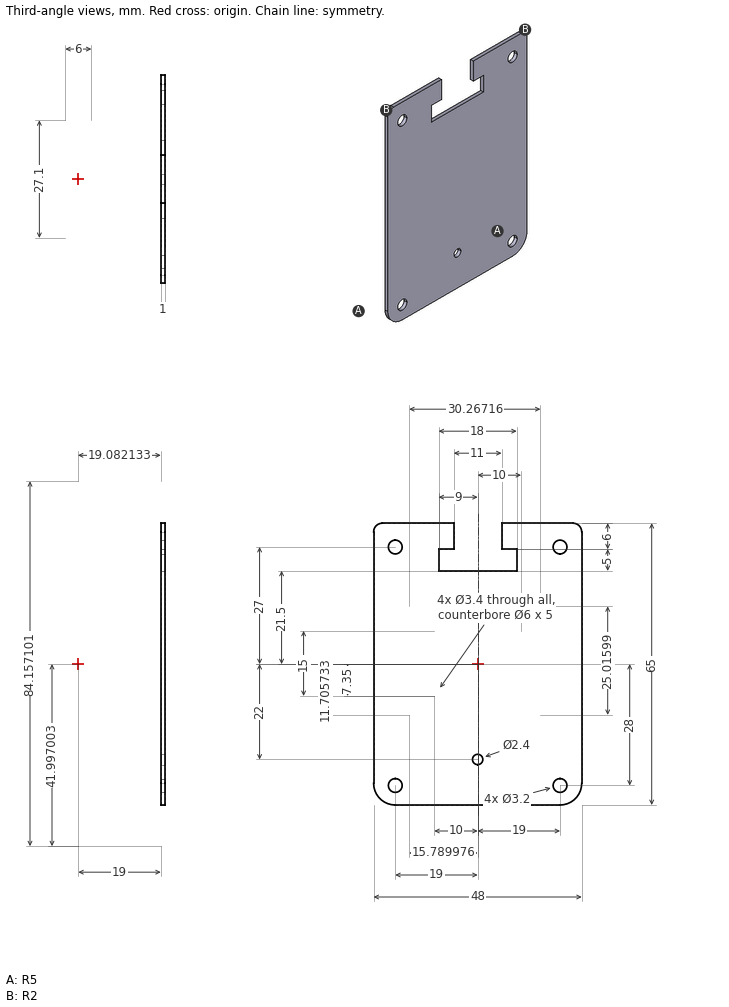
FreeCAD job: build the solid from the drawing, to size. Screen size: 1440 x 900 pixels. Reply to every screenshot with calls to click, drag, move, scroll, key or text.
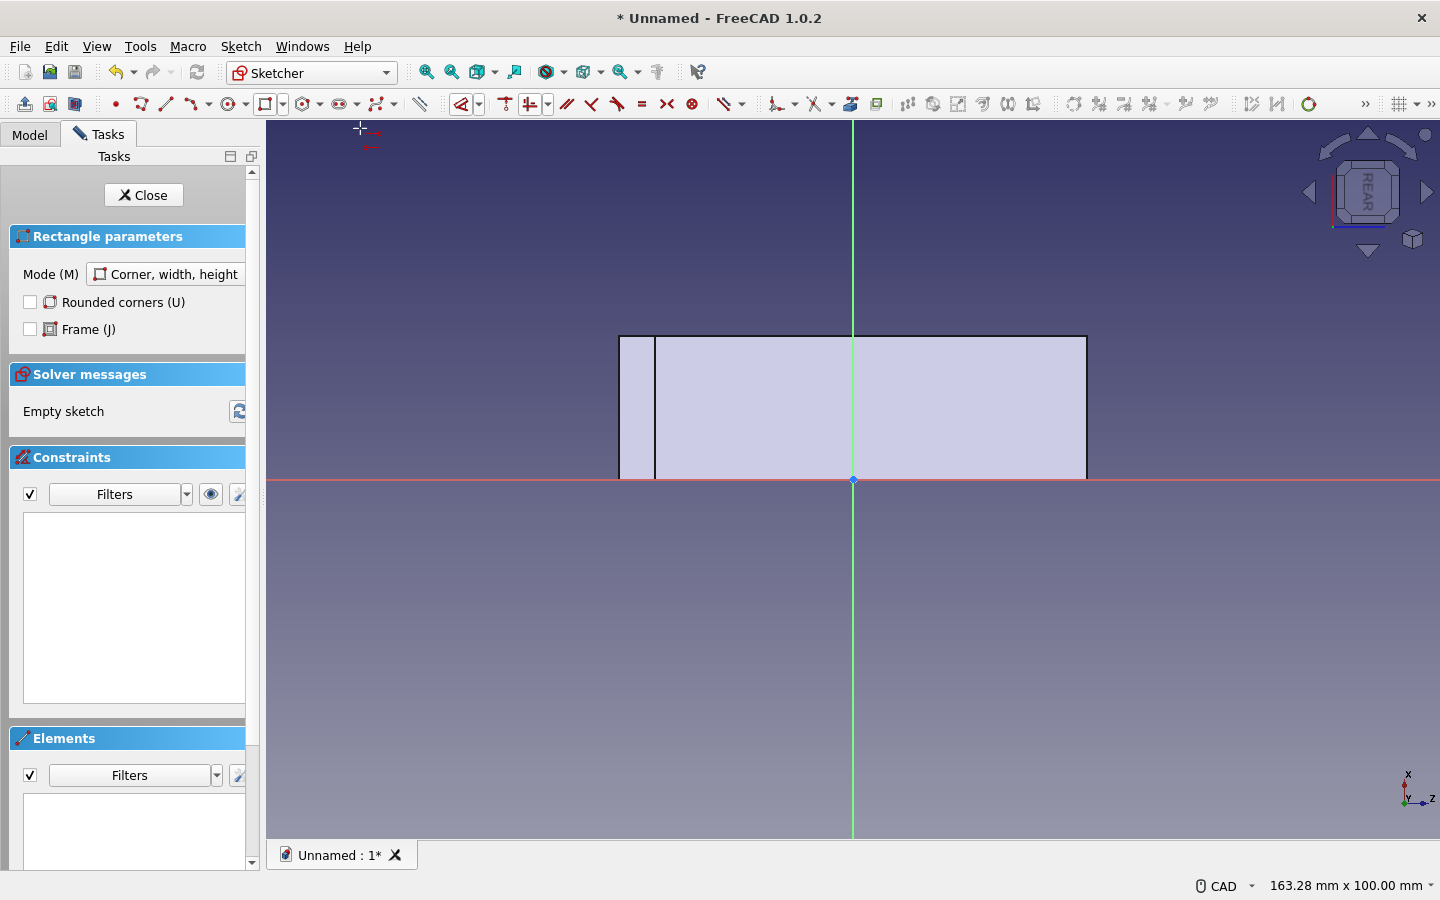
click(551, 343)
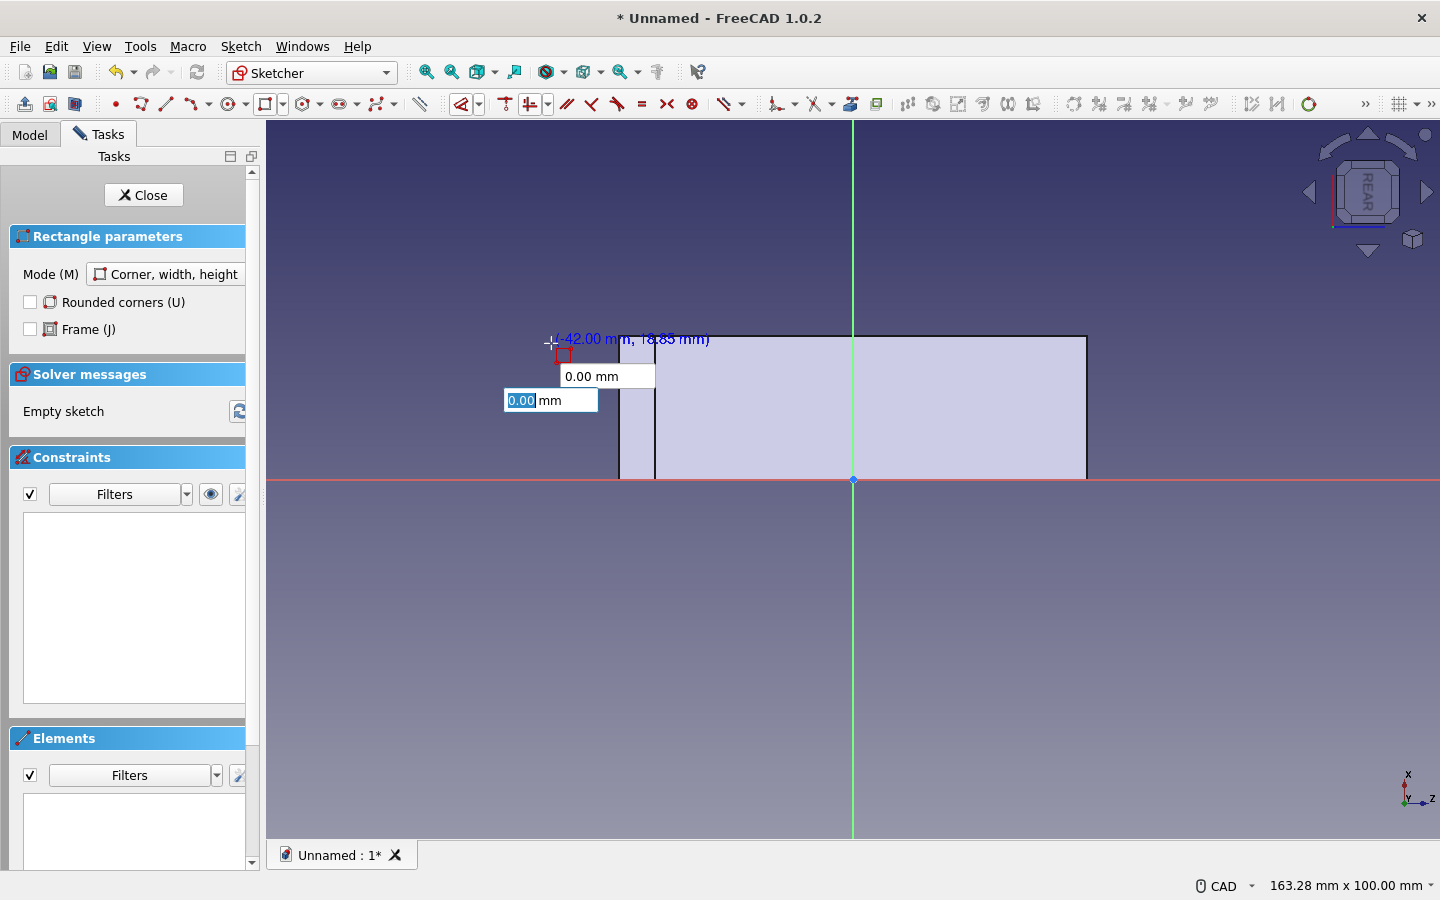
scroll(1156, 480, up, 17)
move(1138, 468)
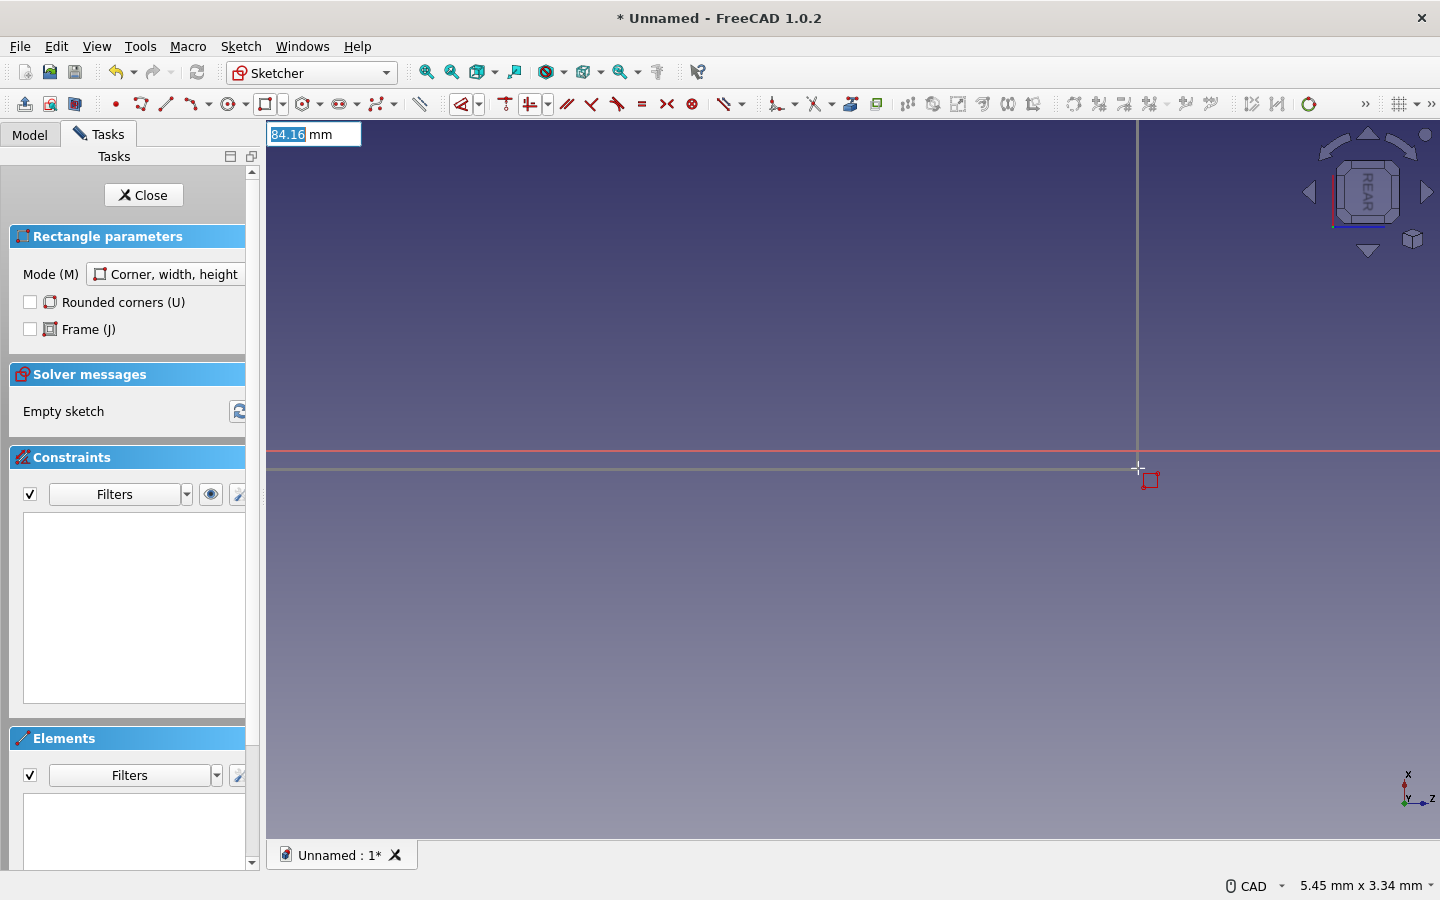
text(84.157101)
key(Tab)
text(19.082133)
key(Return)
key(Escape)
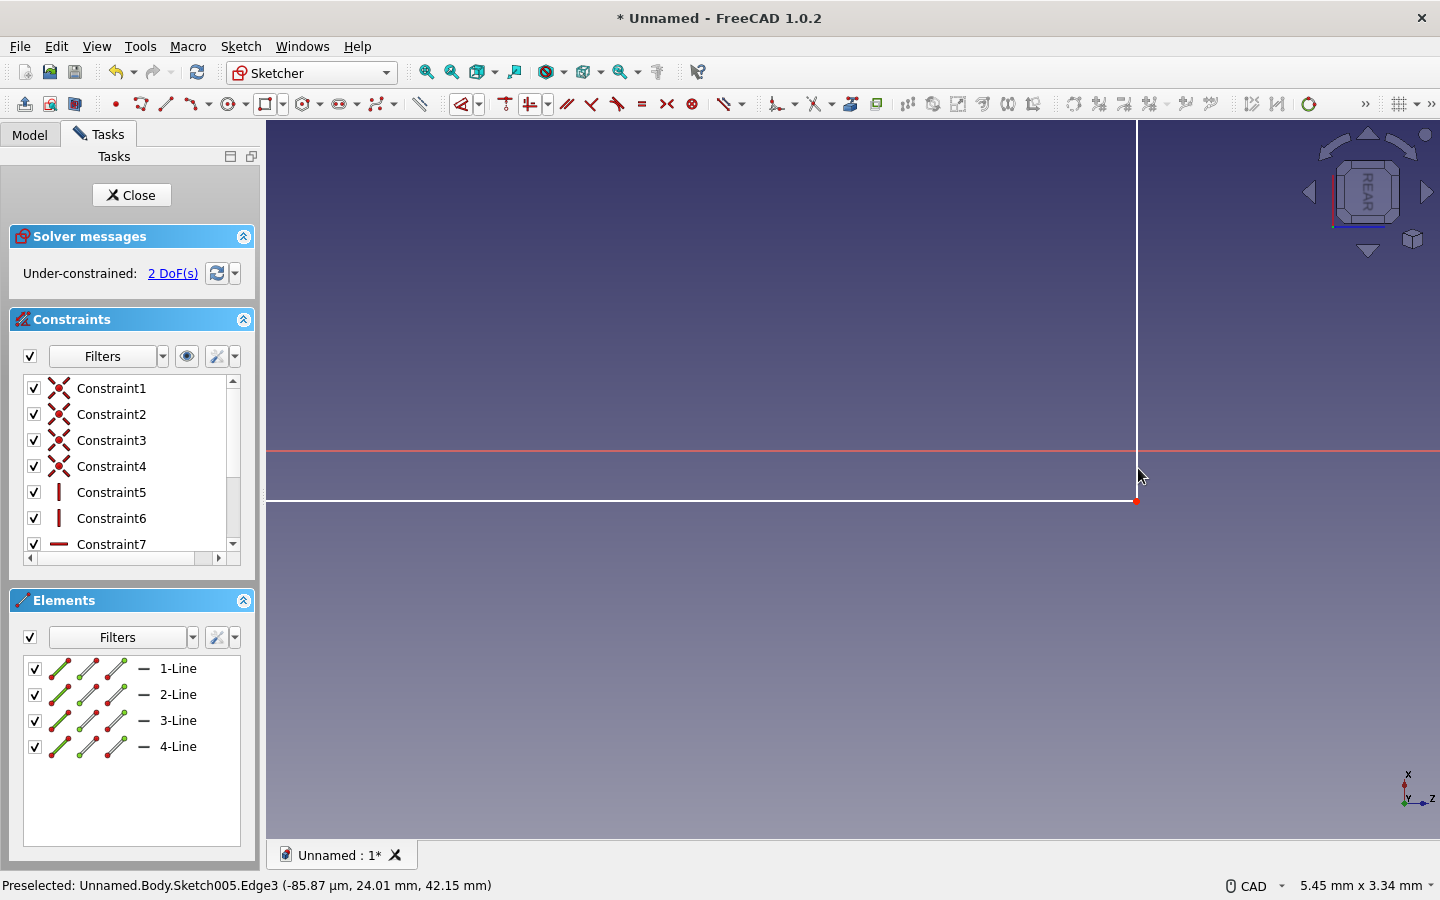
scroll(1241, 588, down, 15)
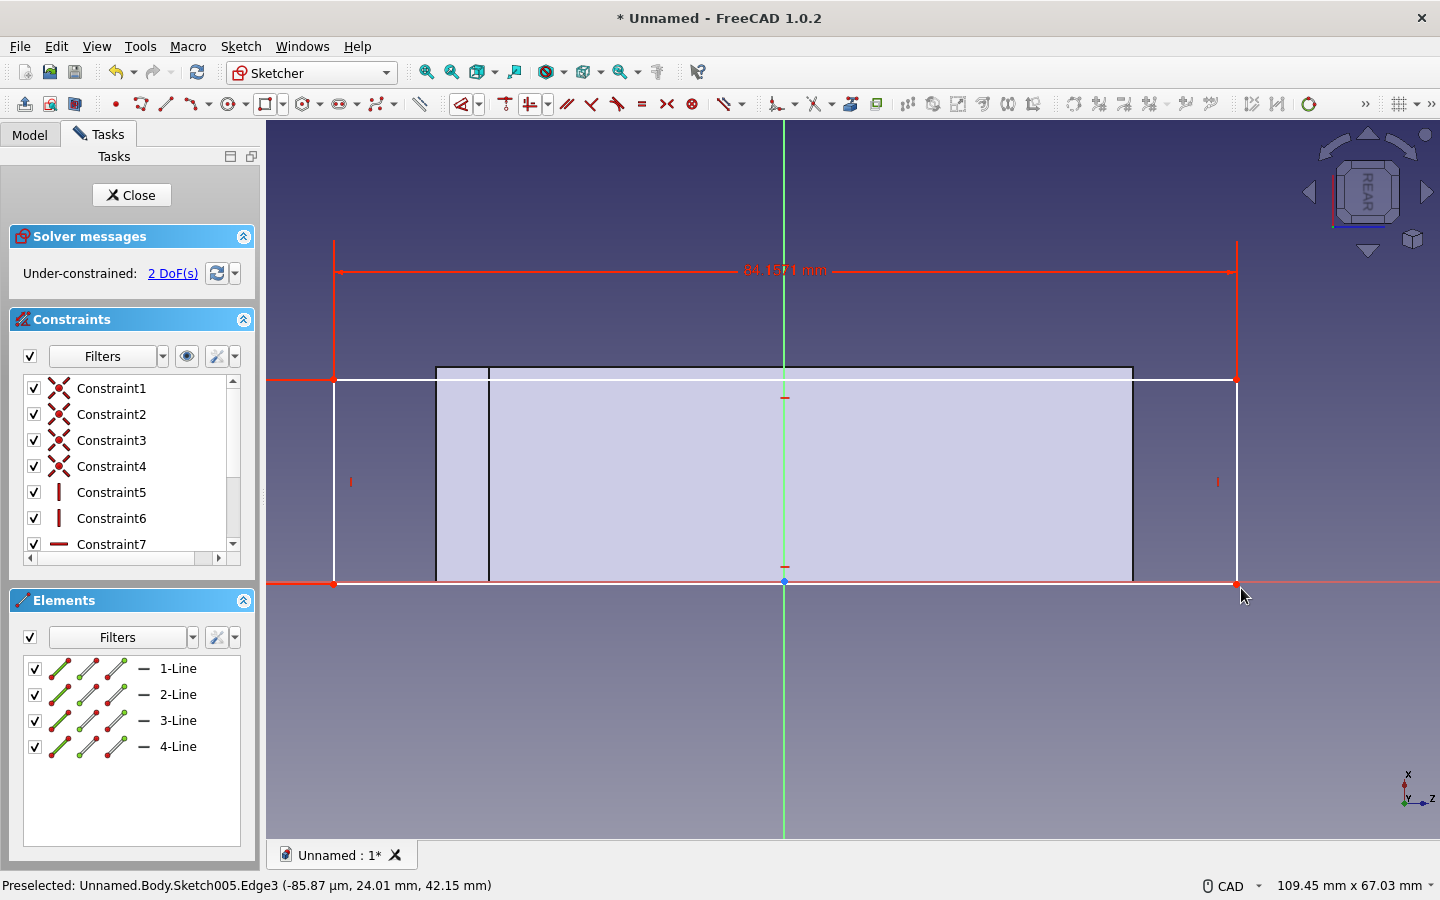
click(334, 380)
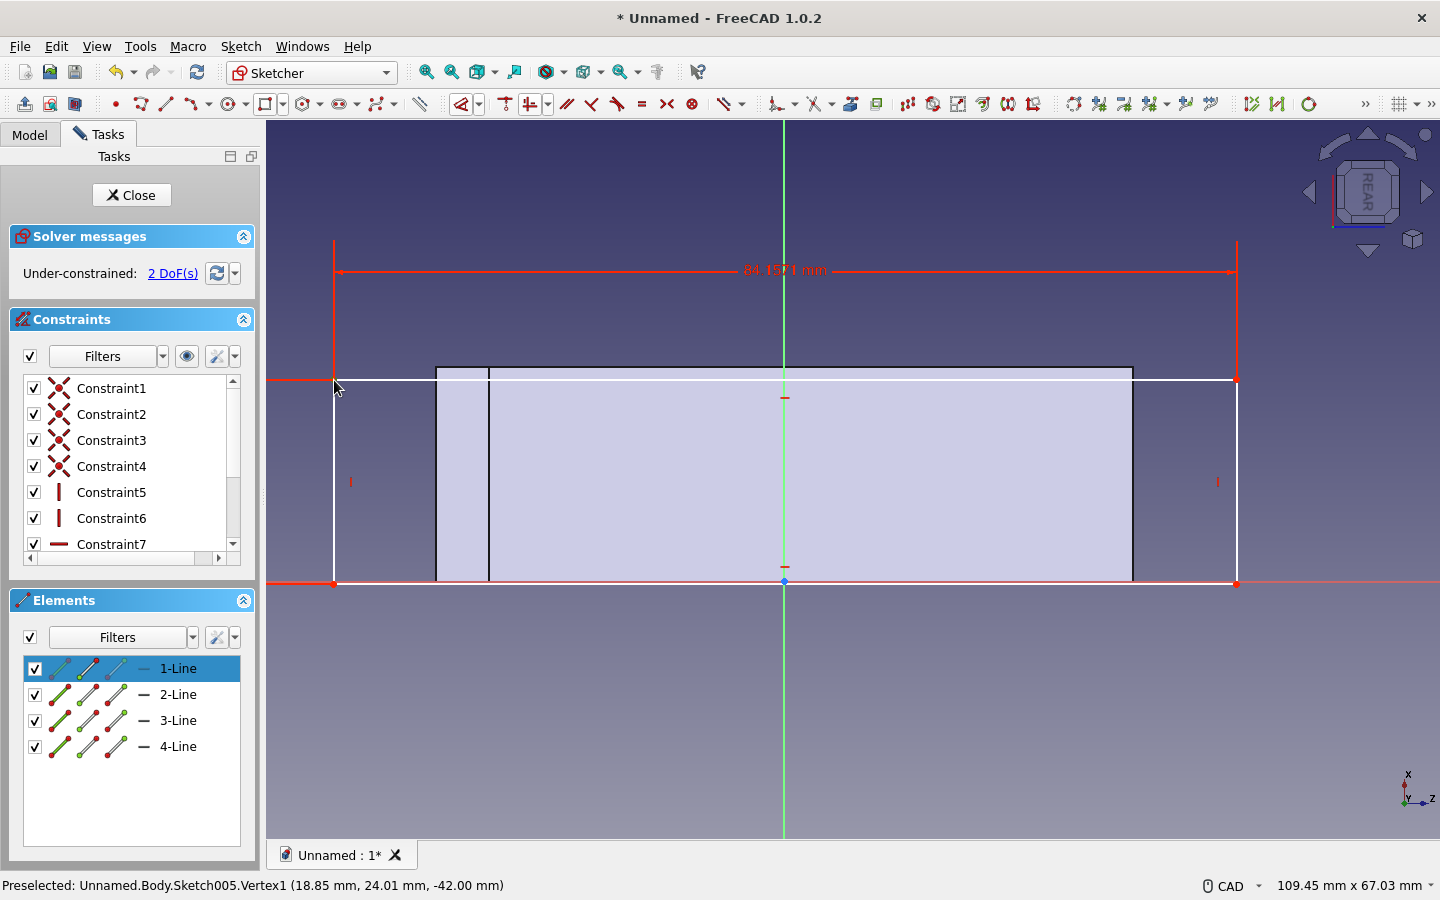
key(i)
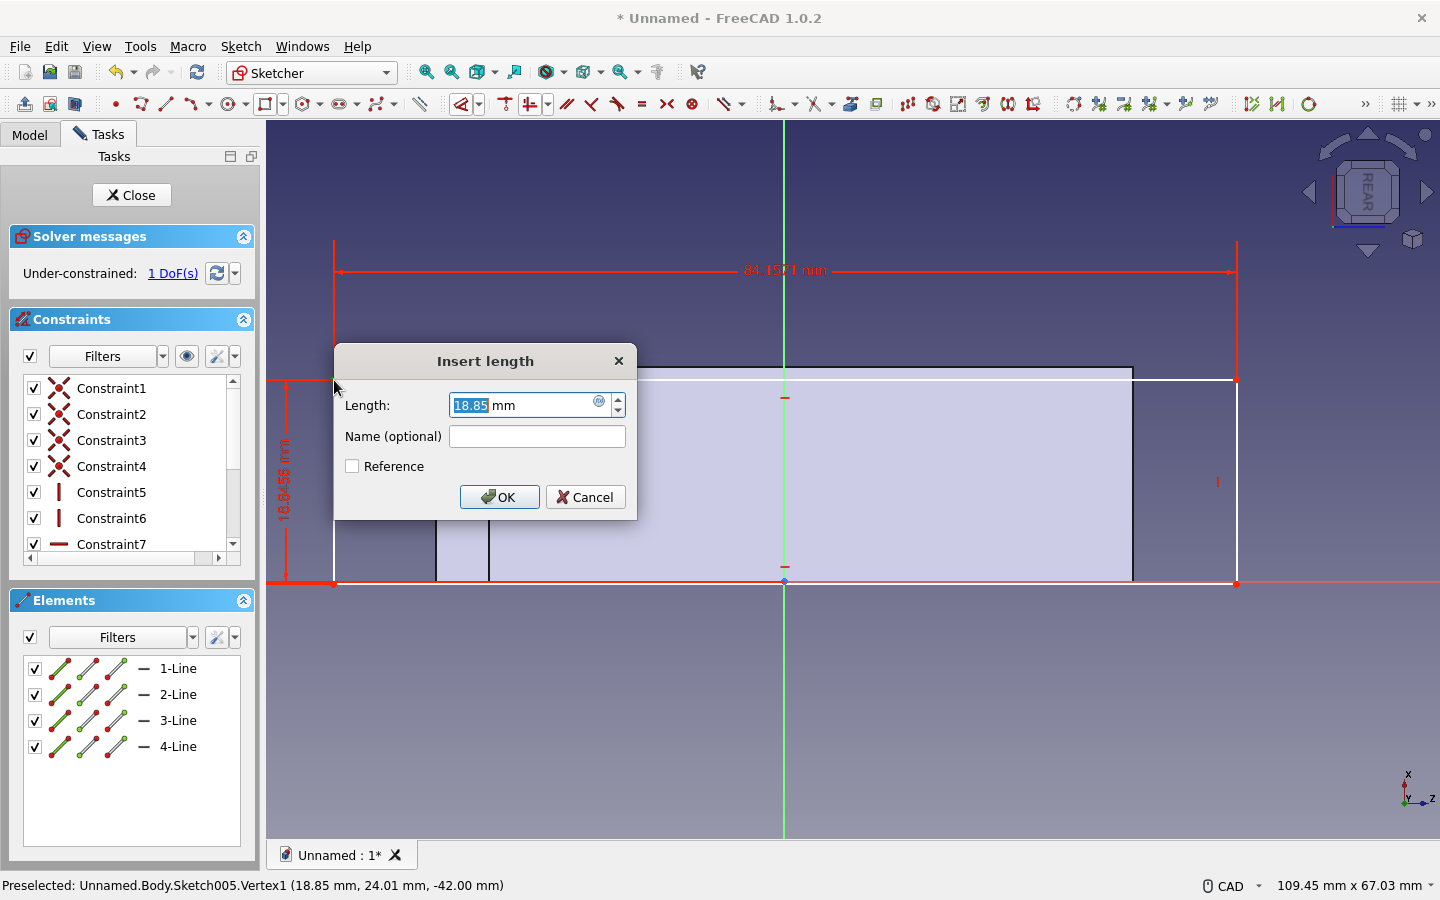
text(19)
key(Return)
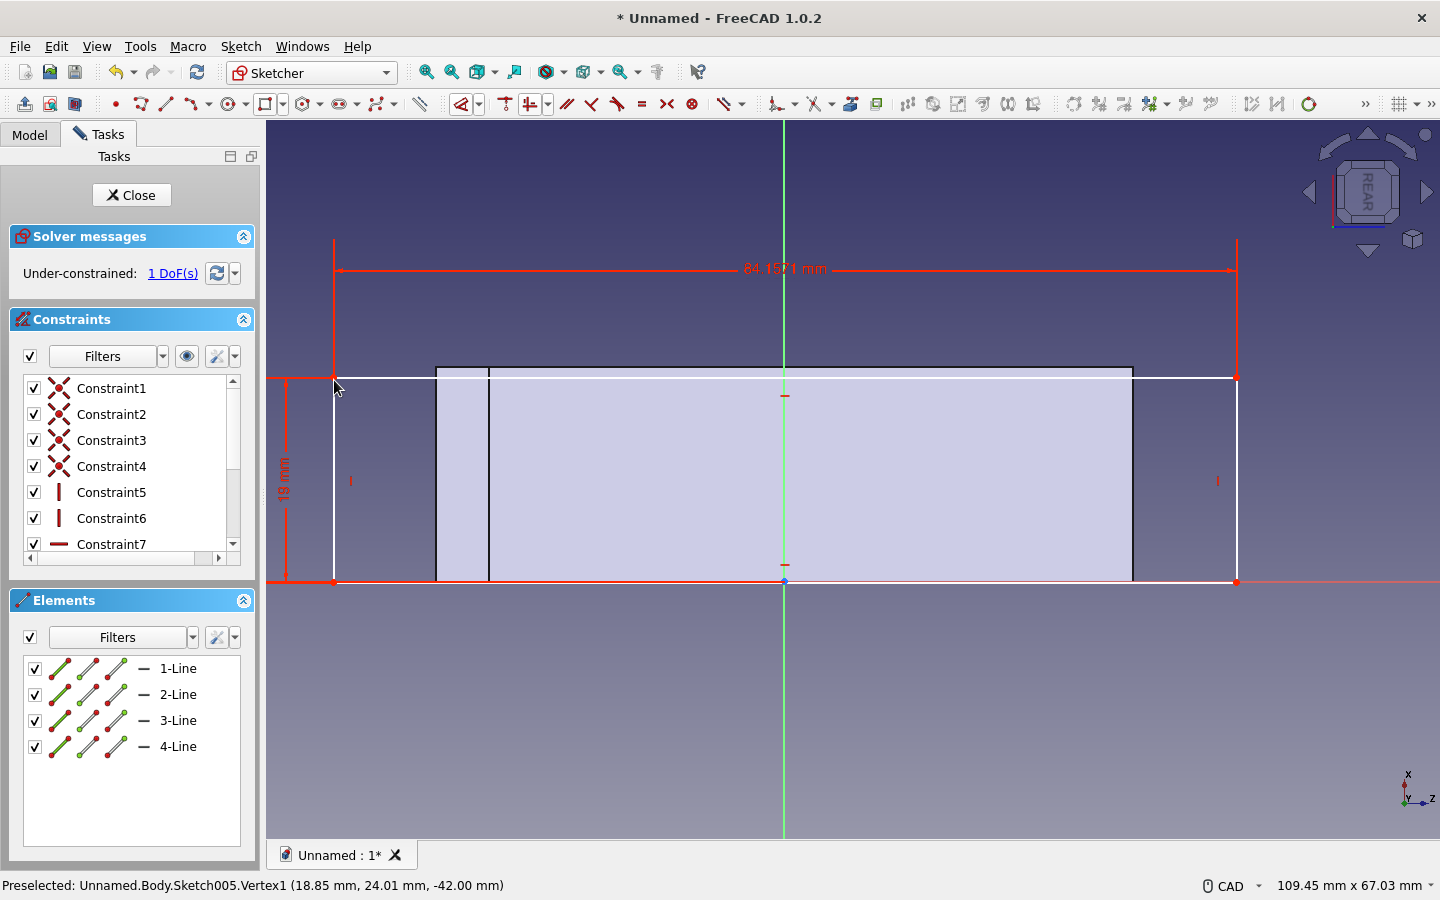
click(334, 378)